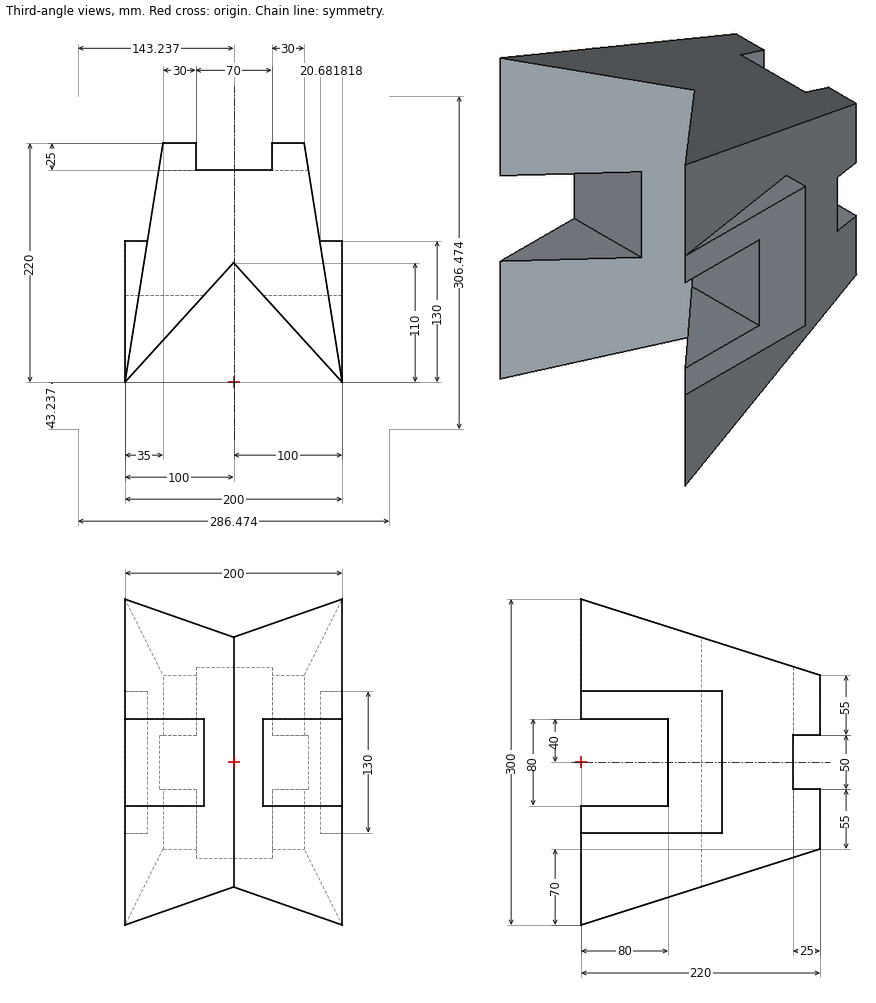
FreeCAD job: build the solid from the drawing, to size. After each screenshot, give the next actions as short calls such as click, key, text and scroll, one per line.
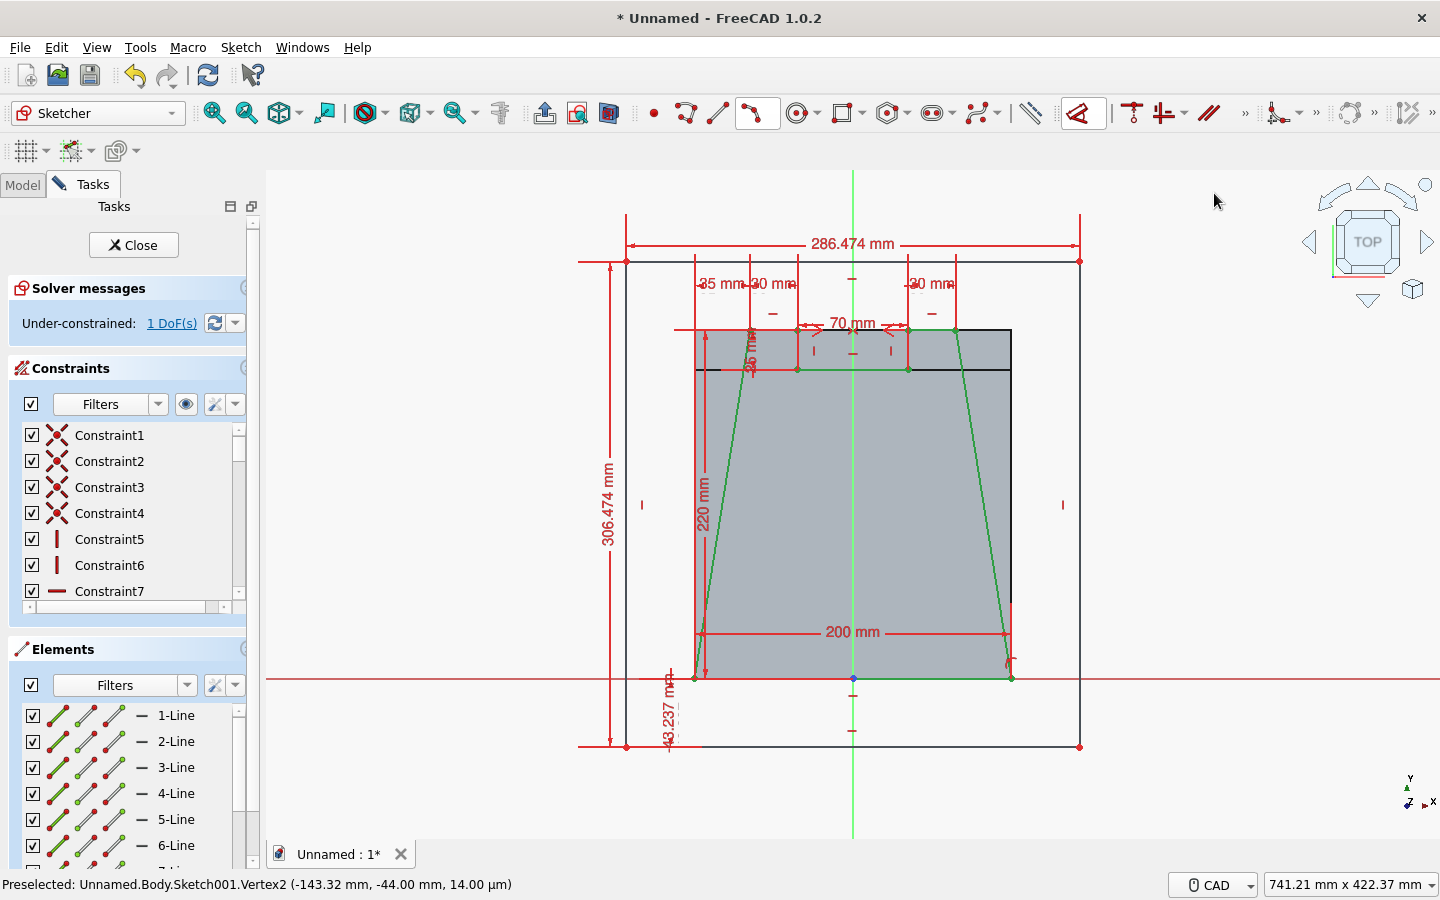
click(626, 262)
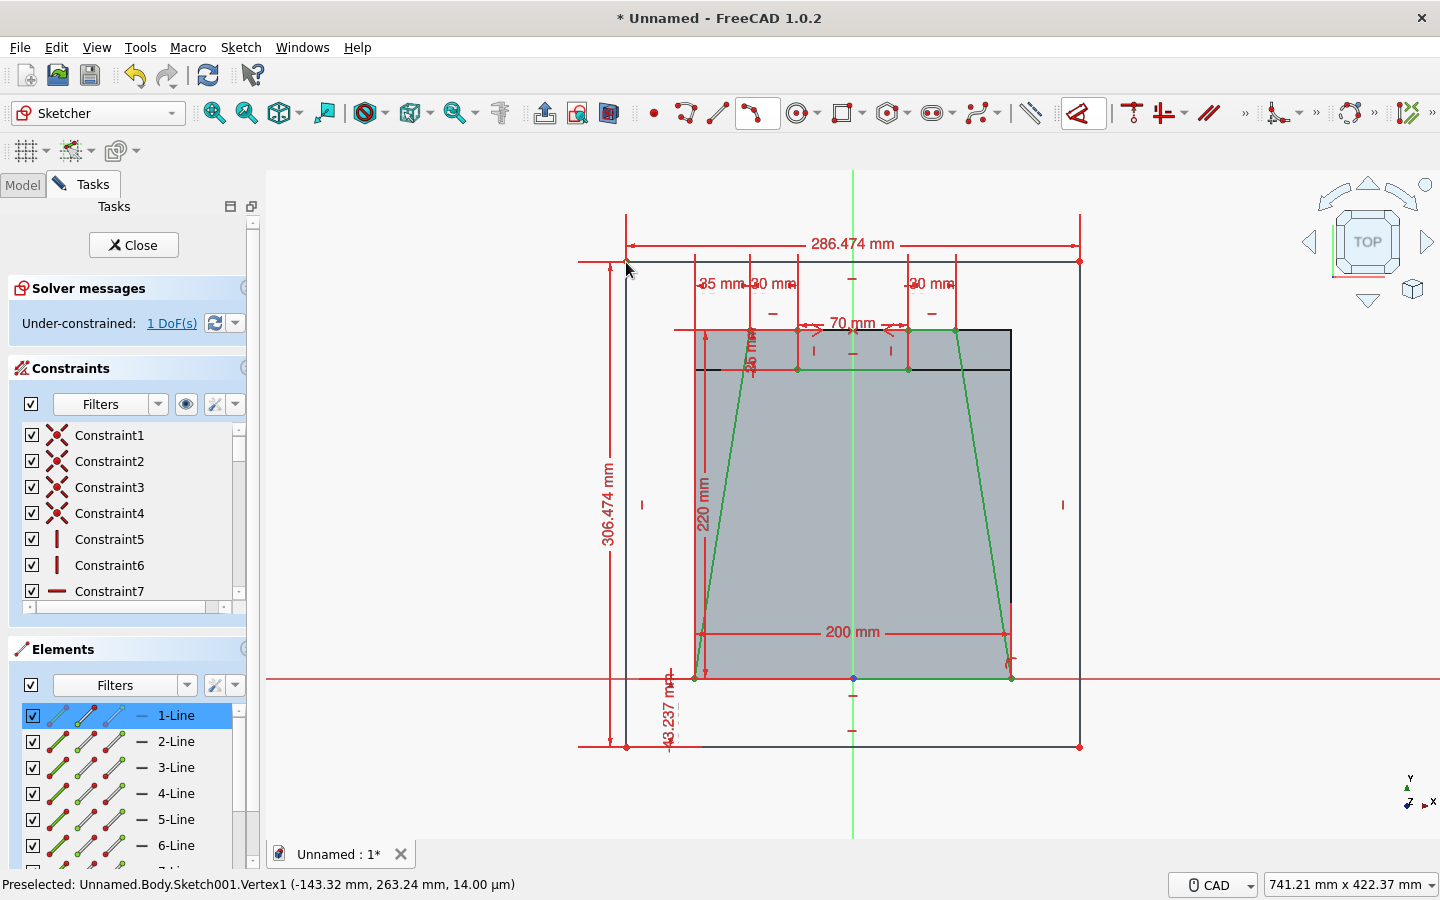
key(l)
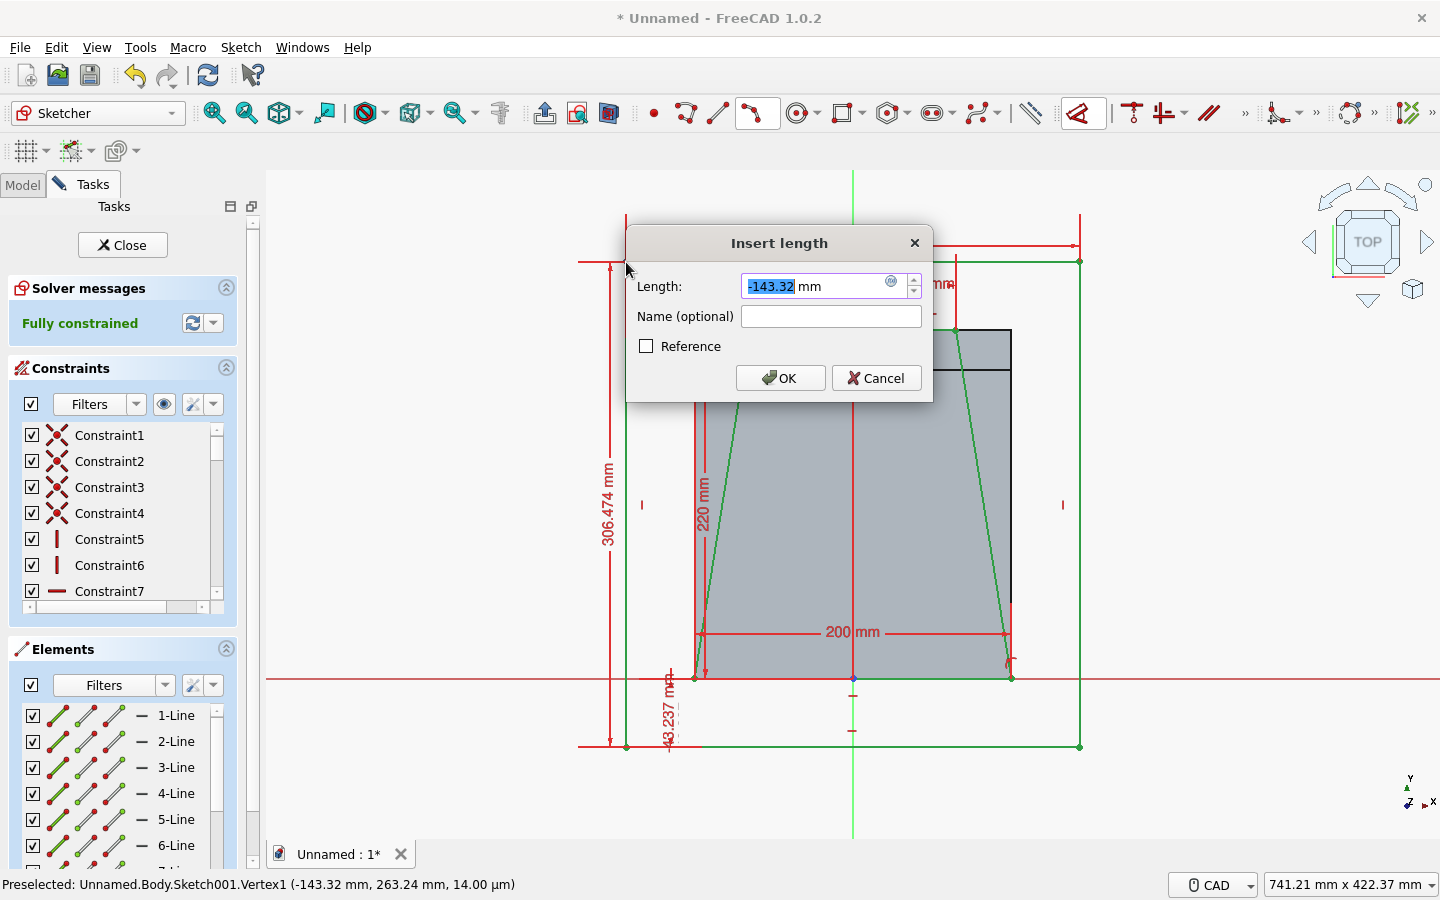
text(-143.237)
key(Return)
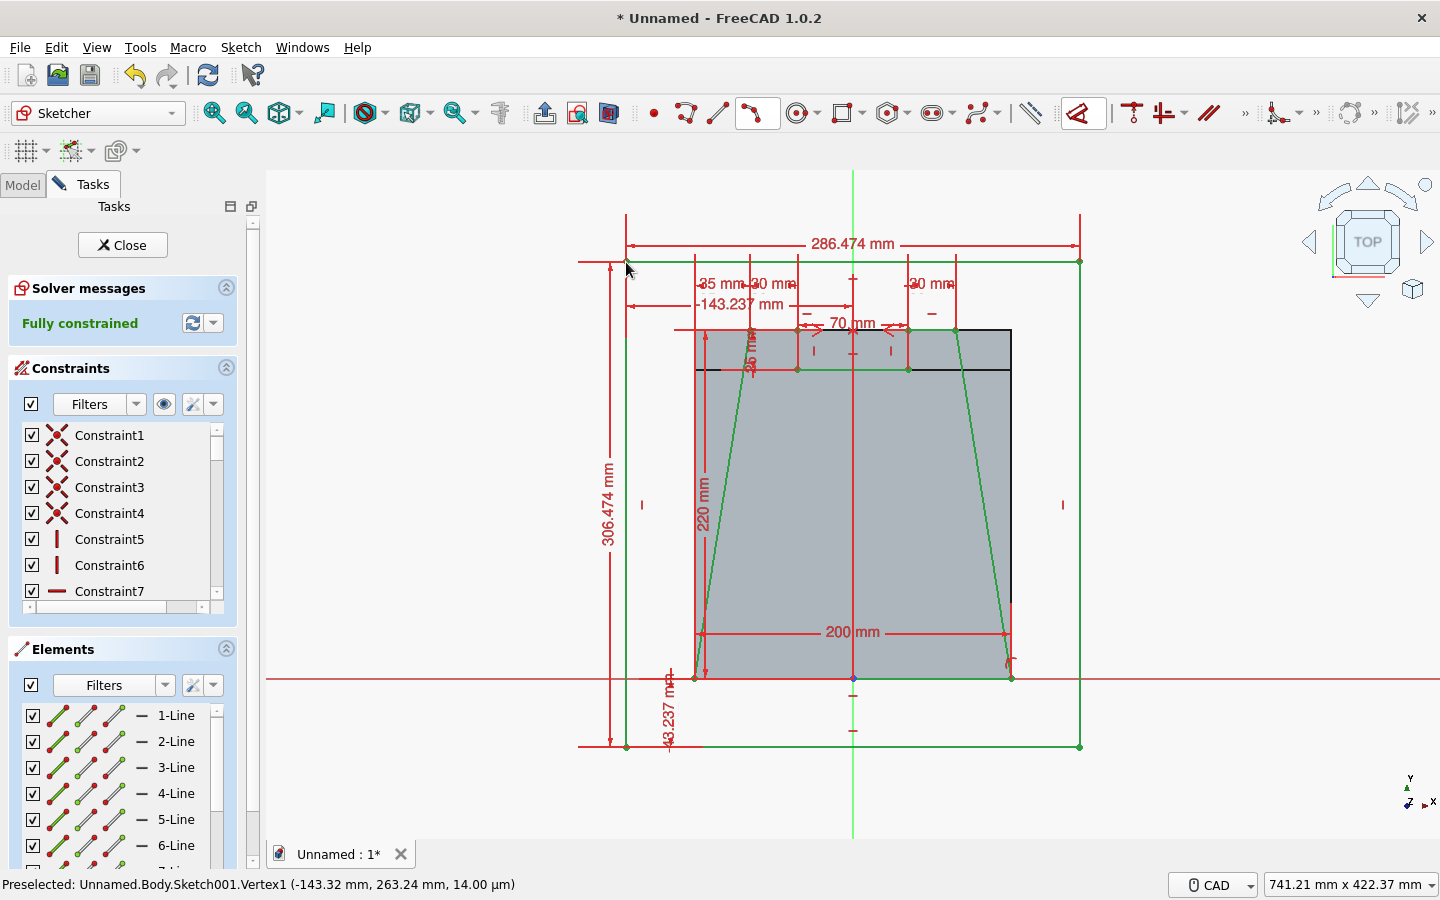
click(123, 245)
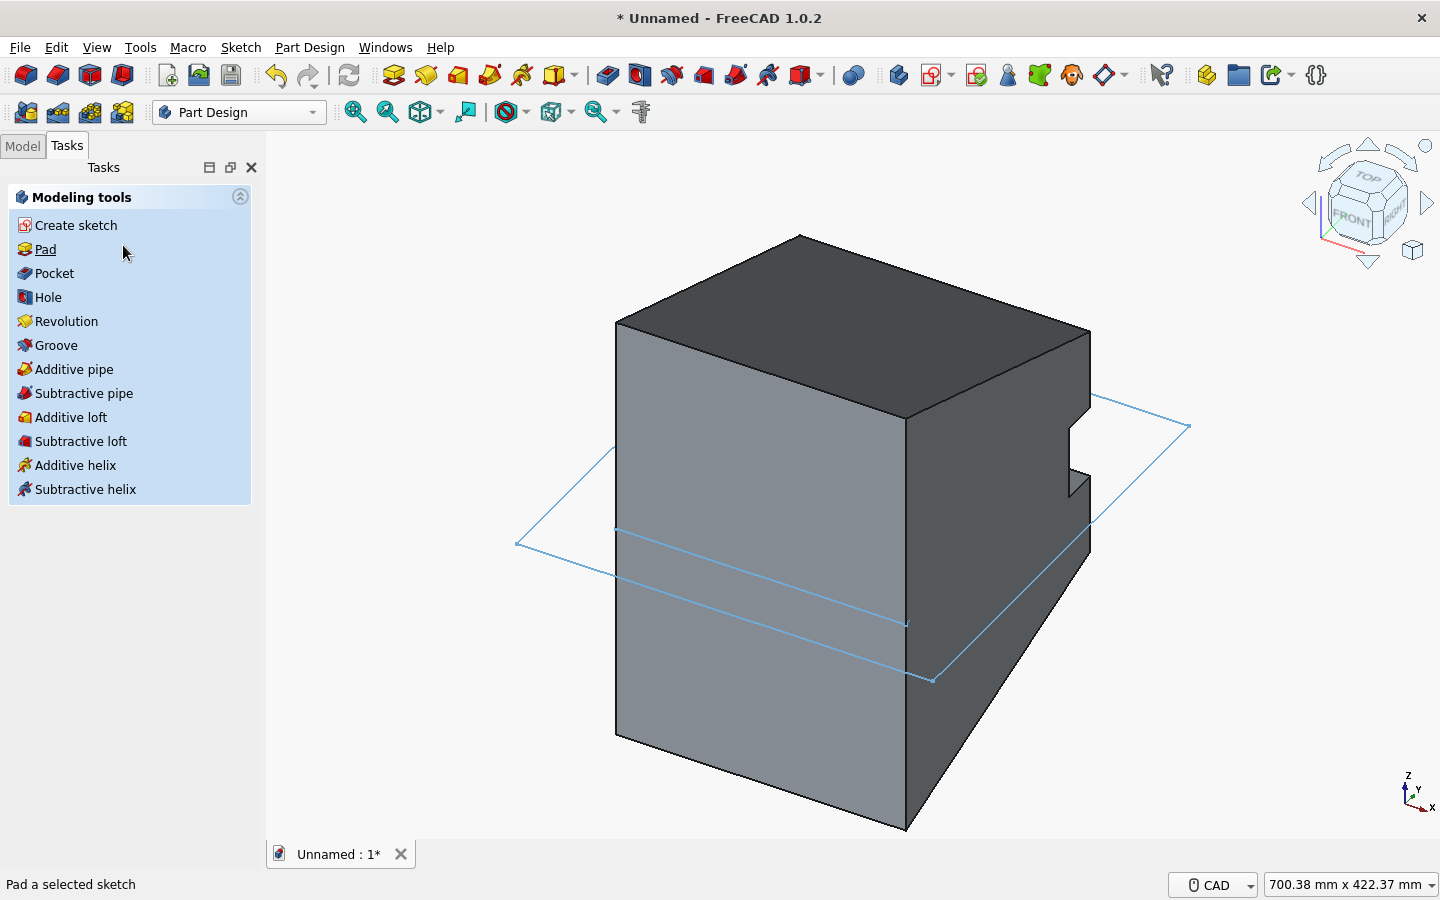
click(608, 76)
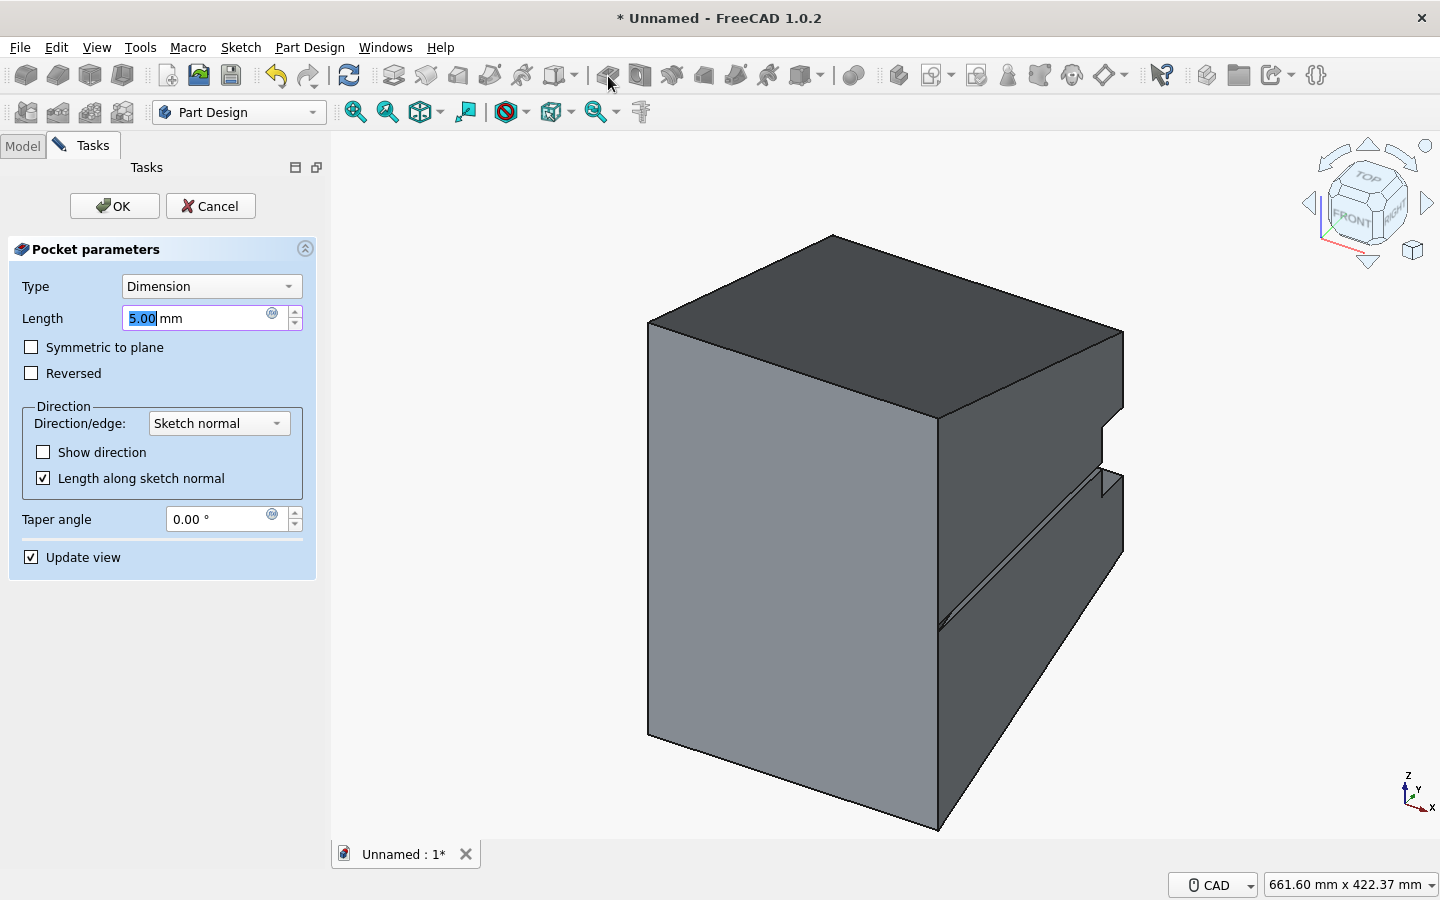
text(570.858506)
key(Tab)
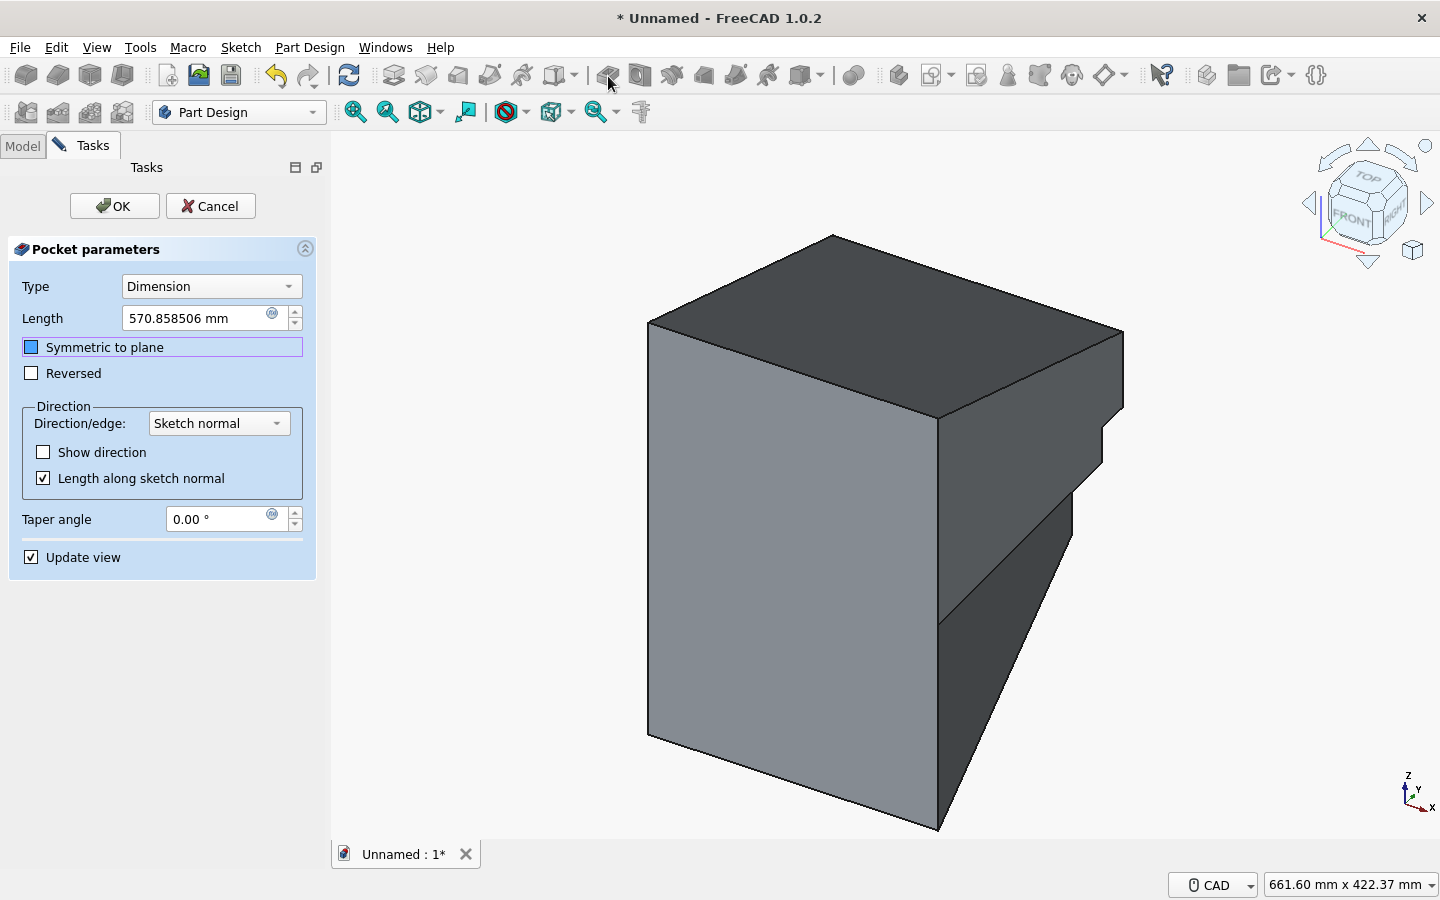
click(30, 347)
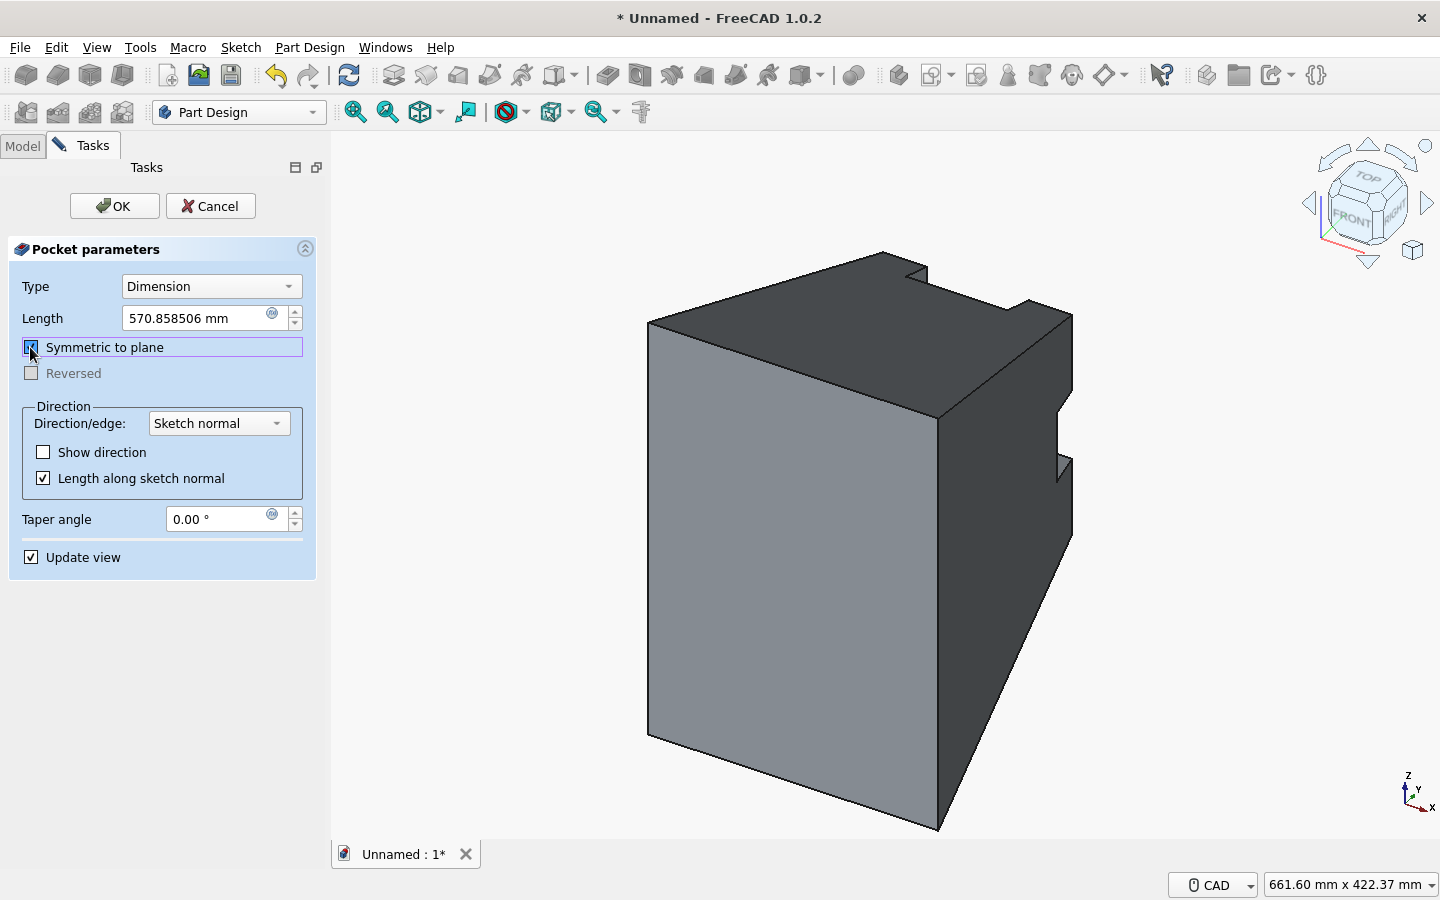
click(115, 206)